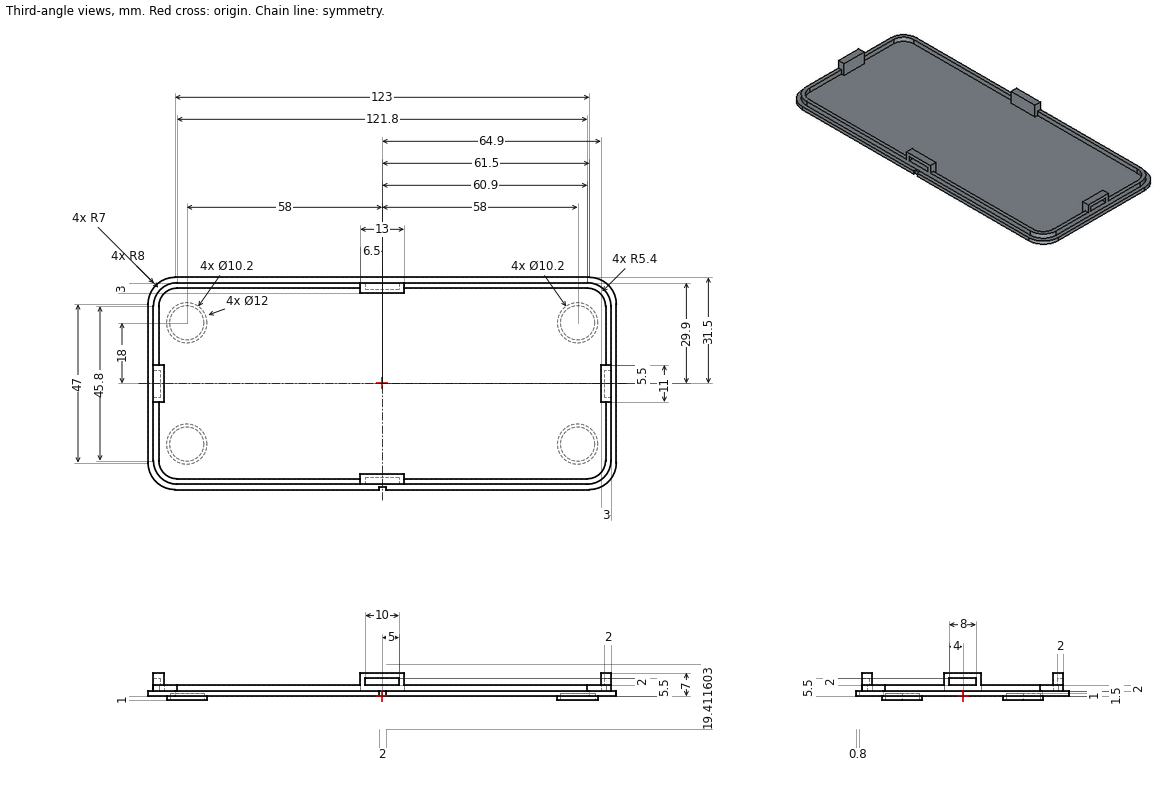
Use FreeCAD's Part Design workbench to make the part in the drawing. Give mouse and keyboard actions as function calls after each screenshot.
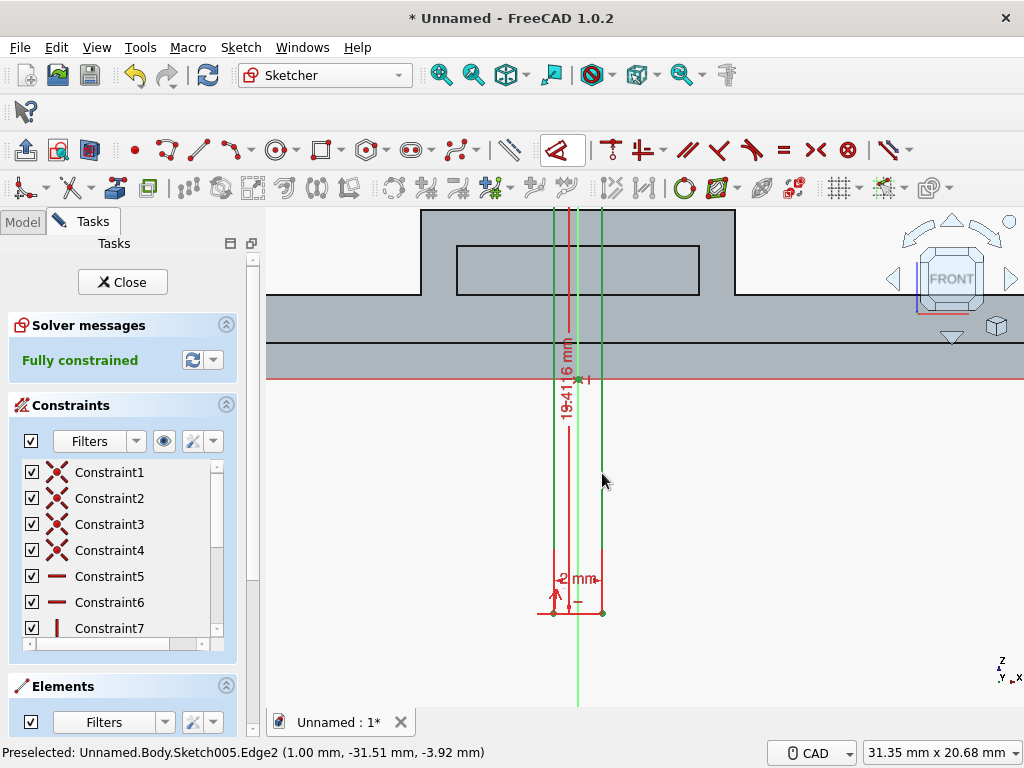
click(123, 282)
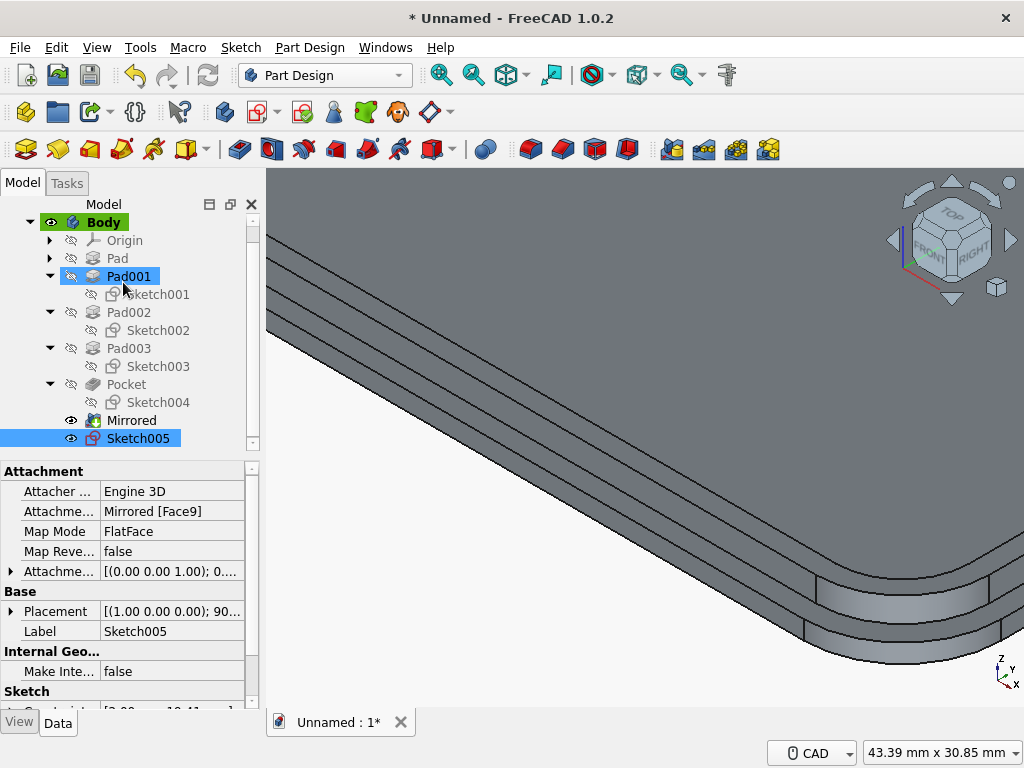
click(240, 150)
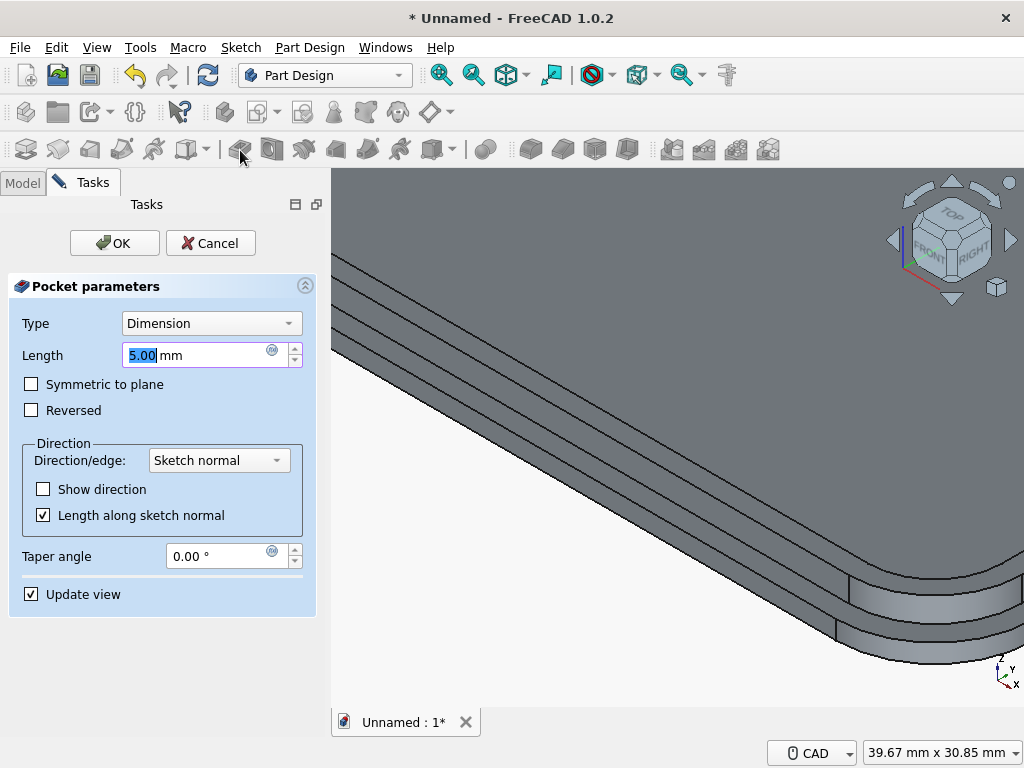
text(0.8)
key(Tab)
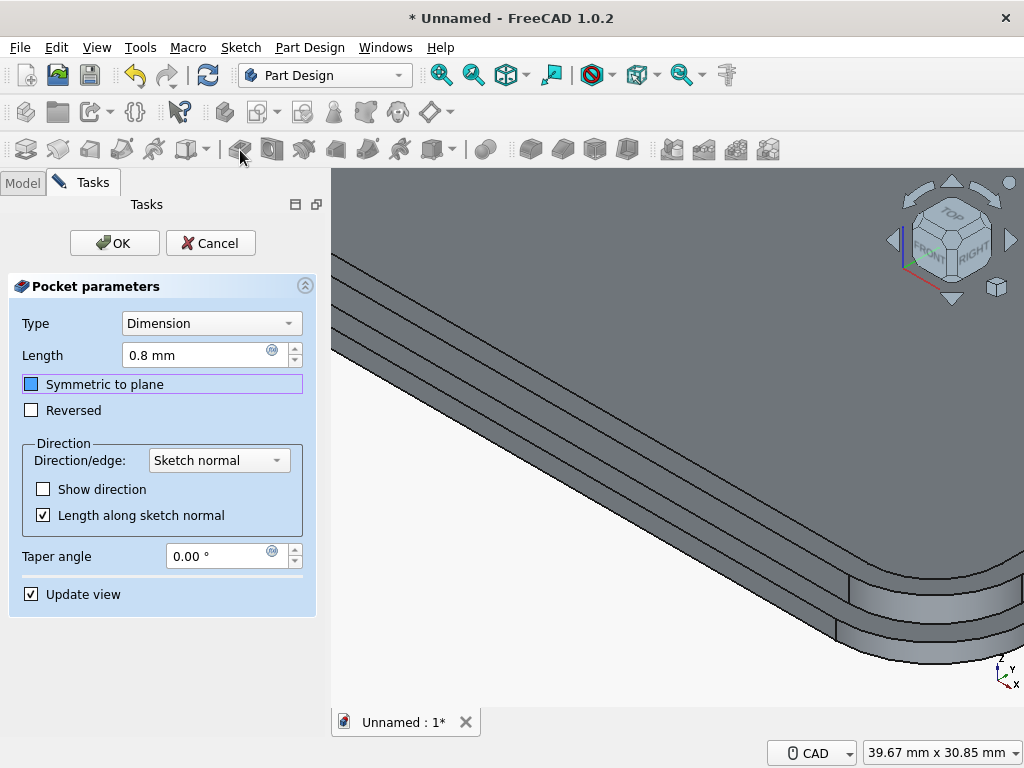
click(115, 243)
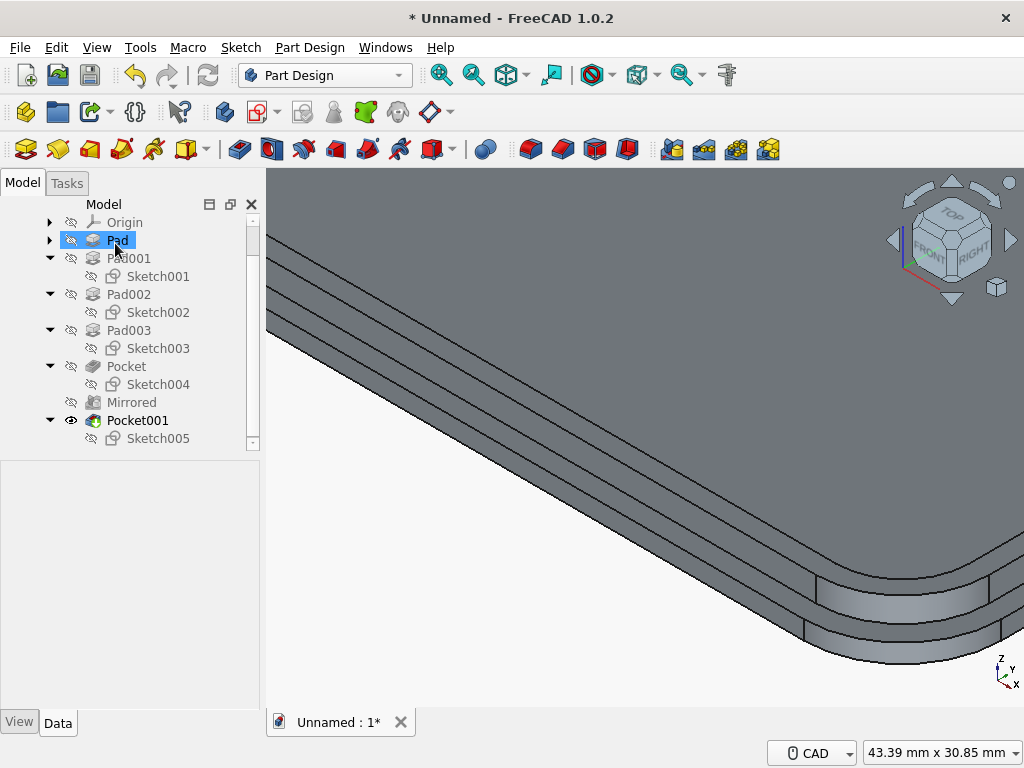
key(v)
key(f)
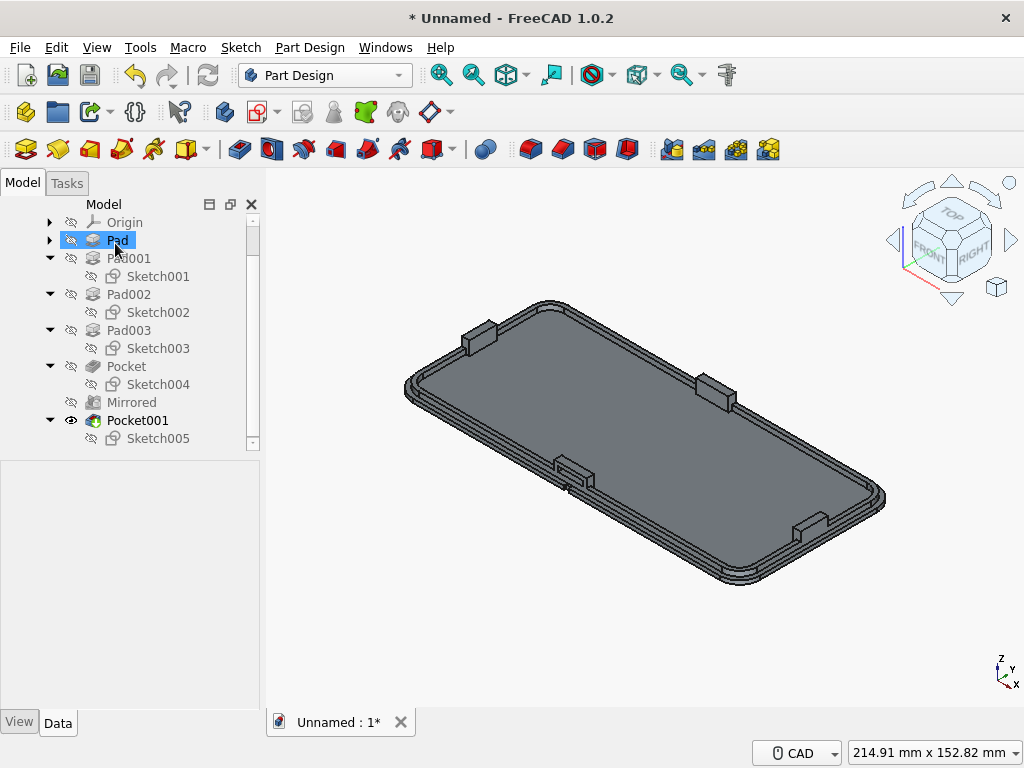
click(50, 222)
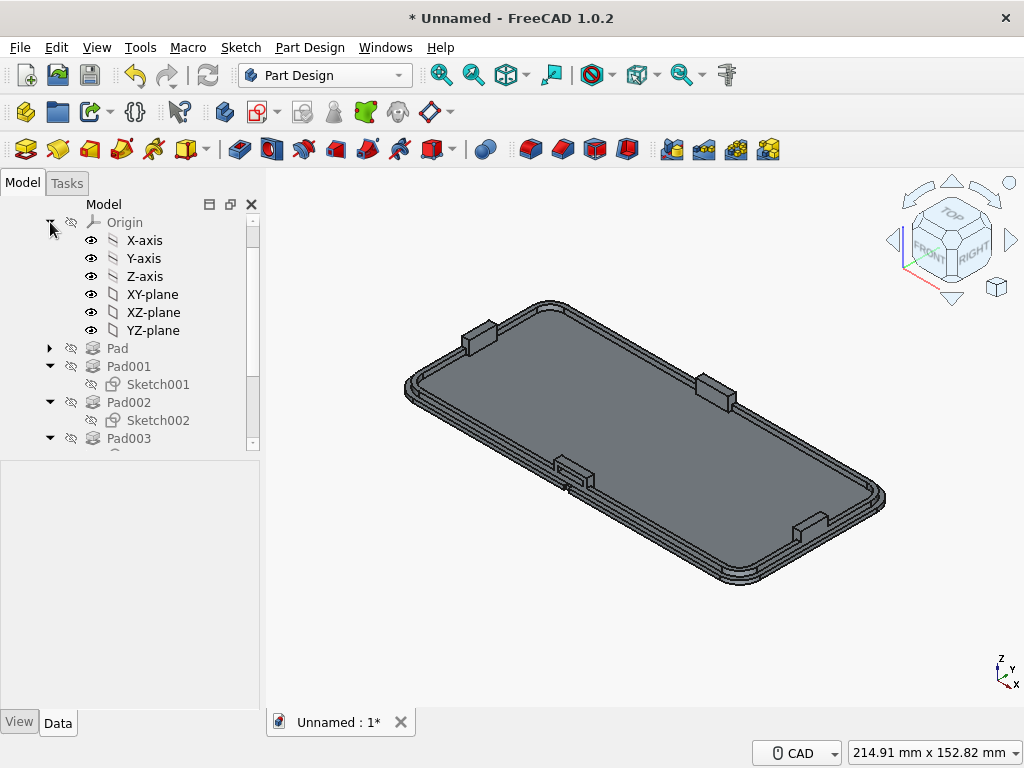
click(136, 294)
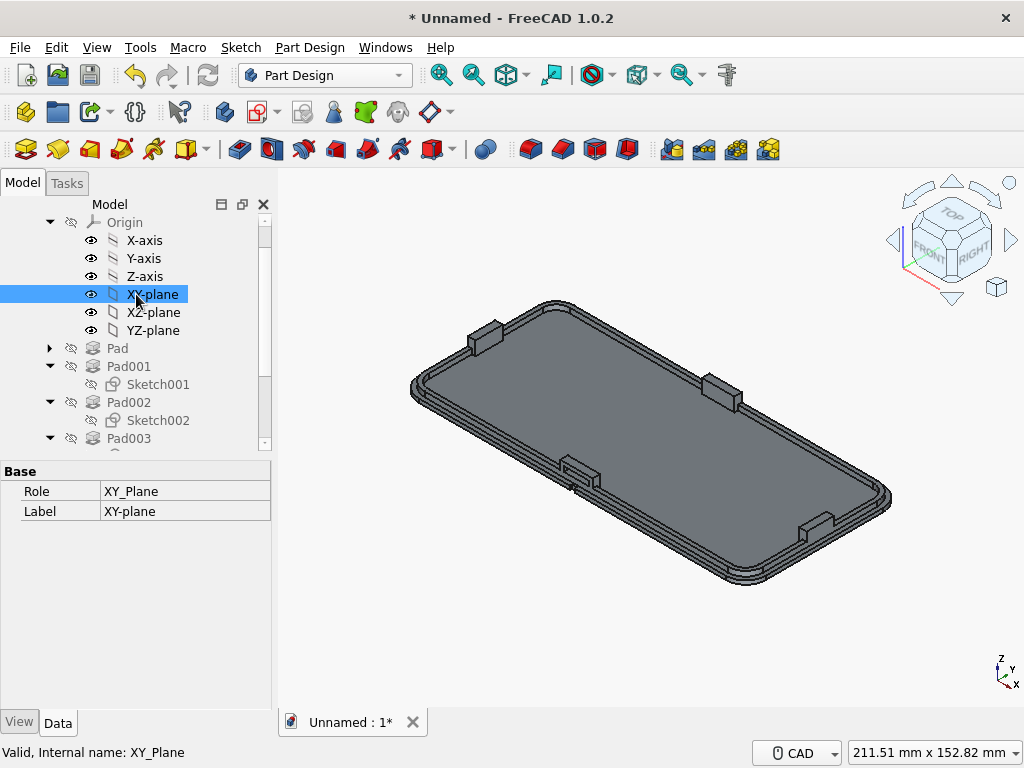
click(430, 112)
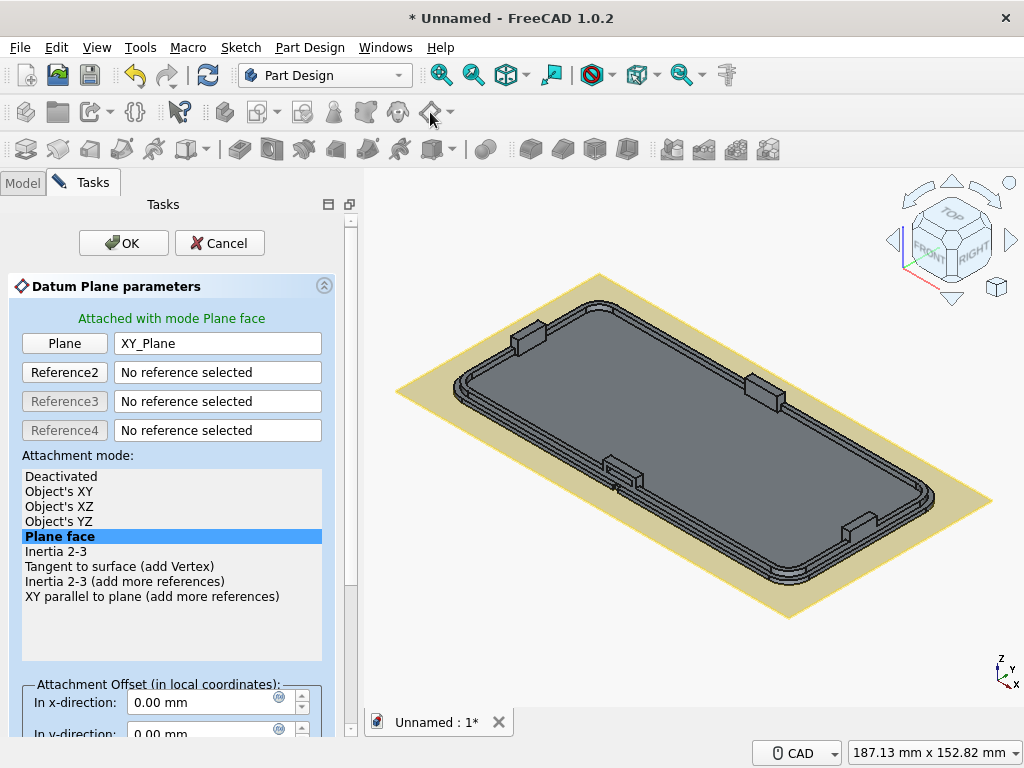
scroll(351, 475, down, 2)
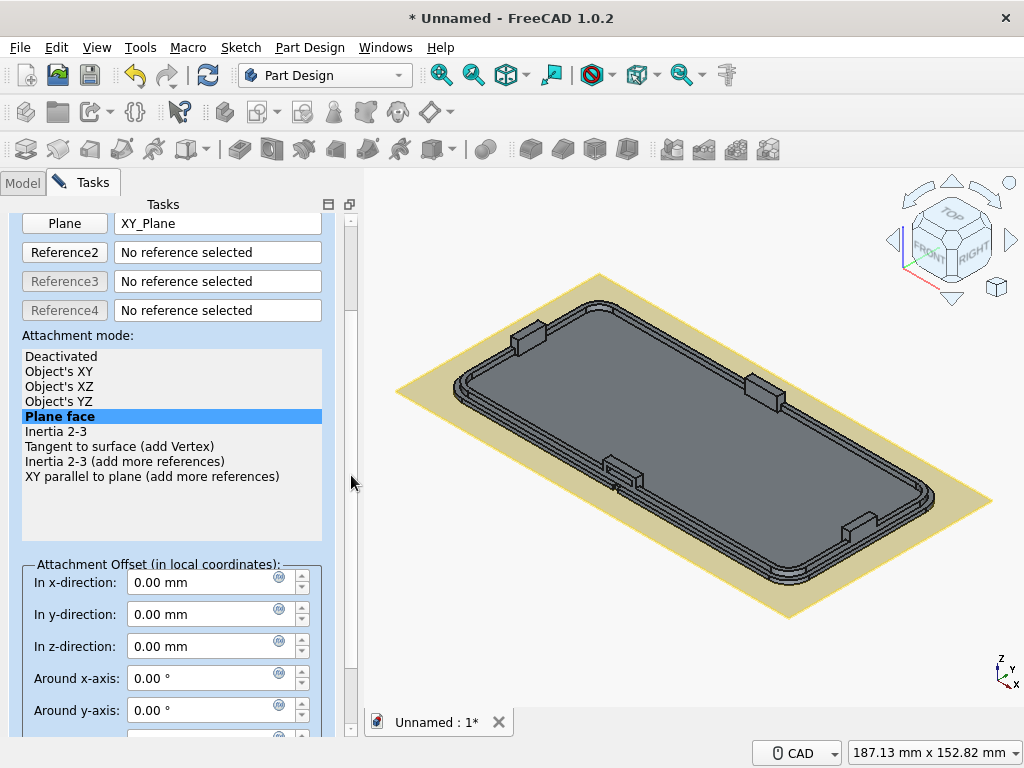
triple_click(210, 646)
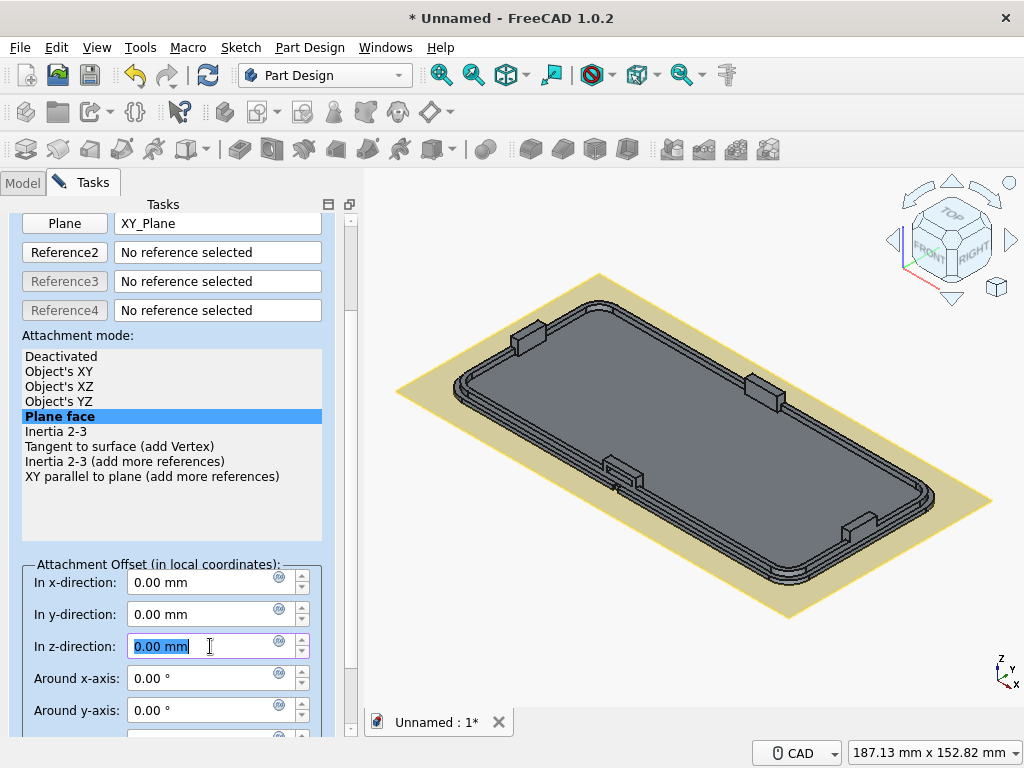
text(1)
key(Tab)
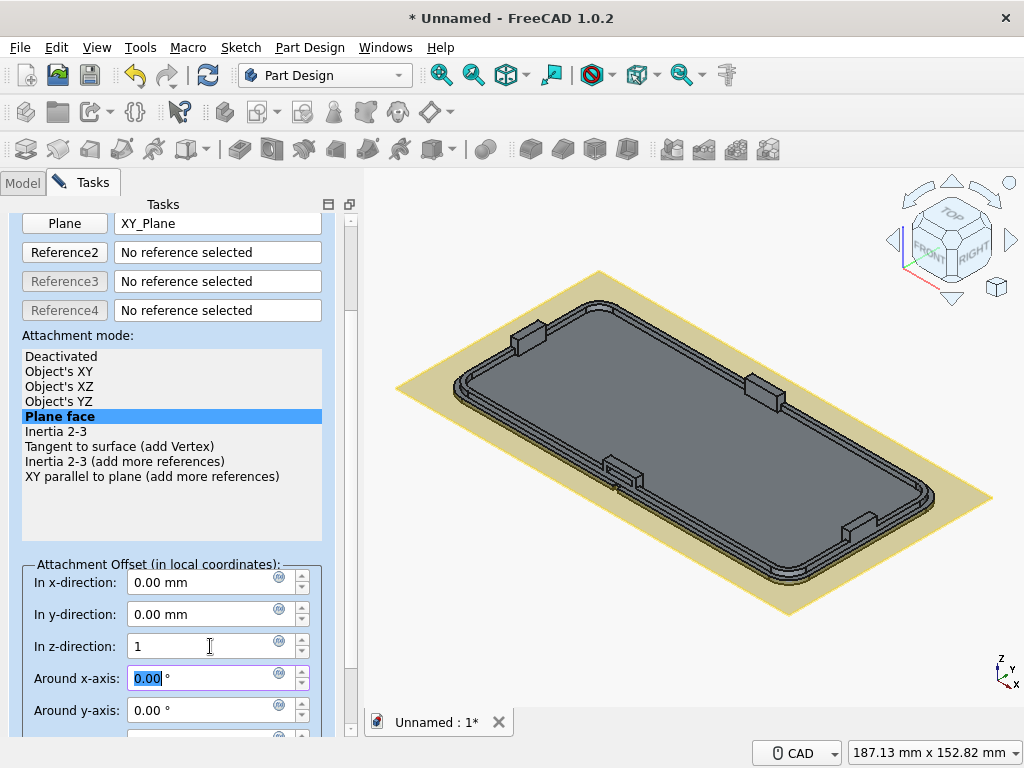
scroll(351, 475, up, 3)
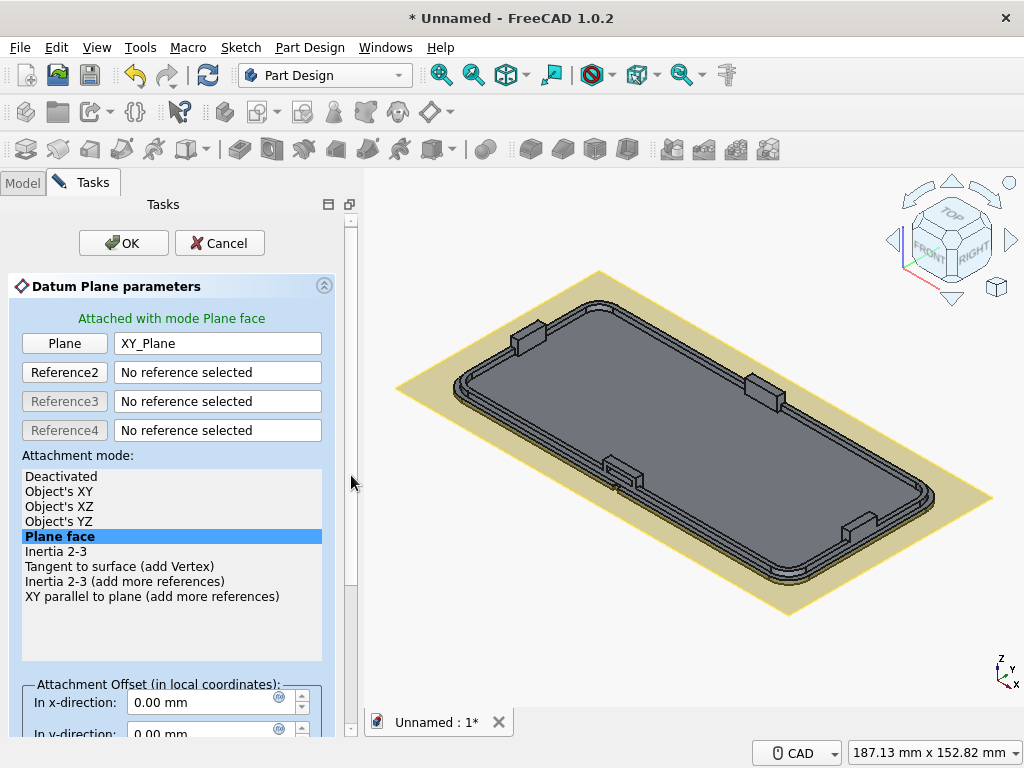
click(124, 243)